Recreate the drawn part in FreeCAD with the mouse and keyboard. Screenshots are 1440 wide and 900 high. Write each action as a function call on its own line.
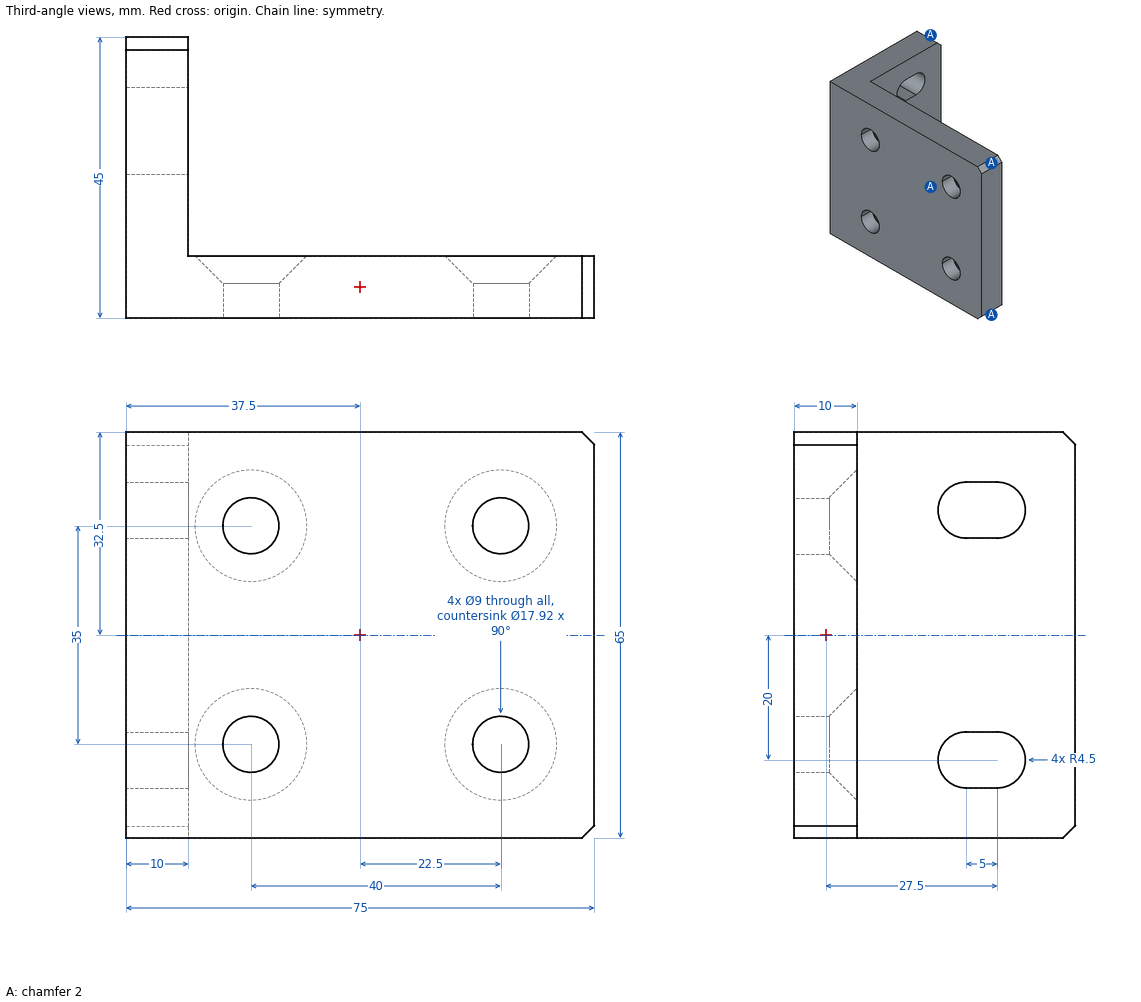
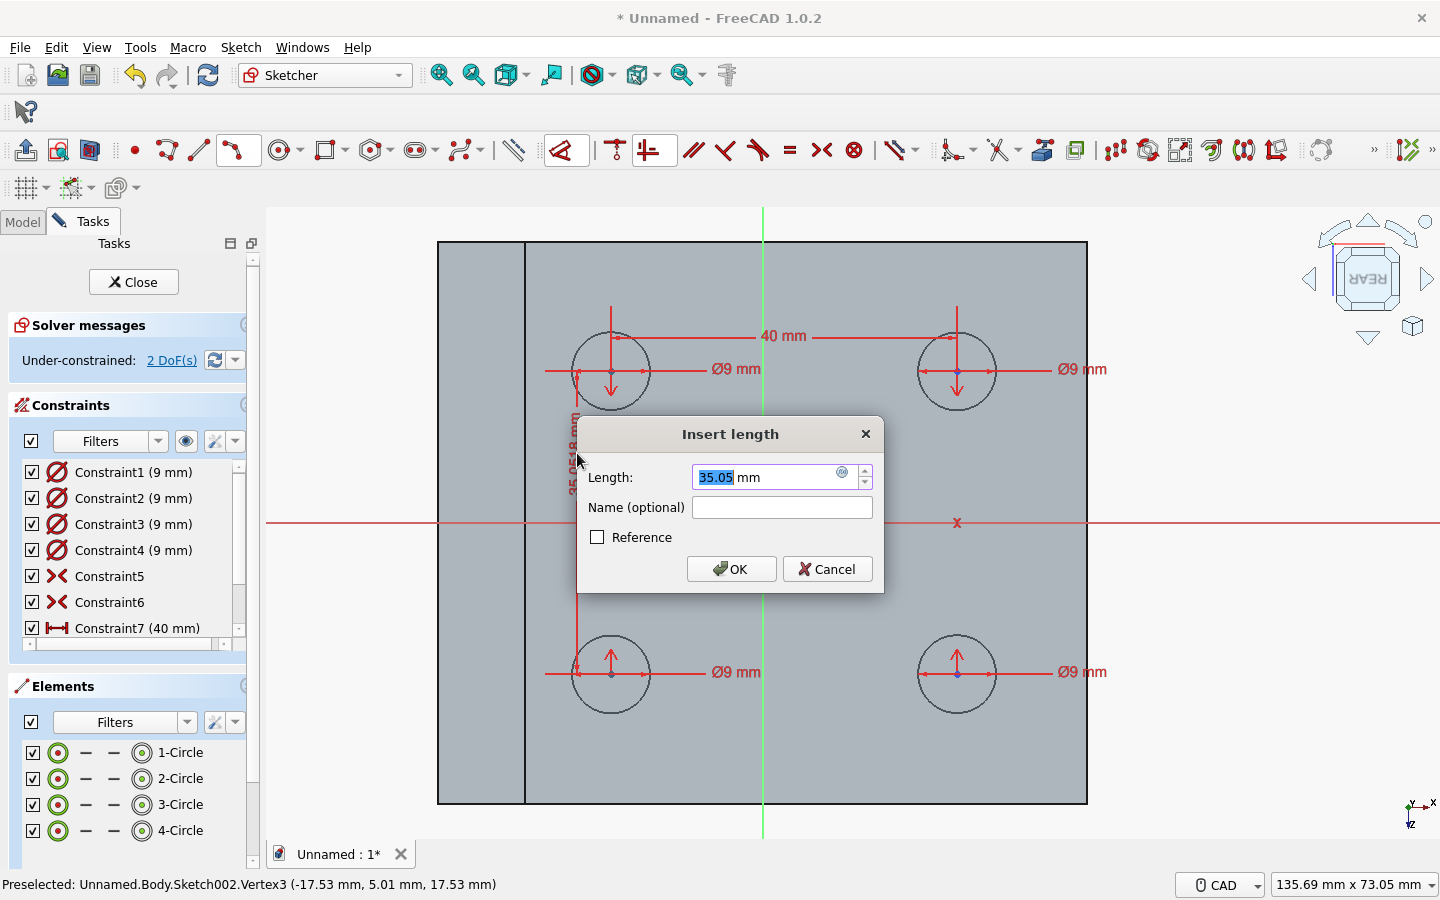
text(35)
key(Return)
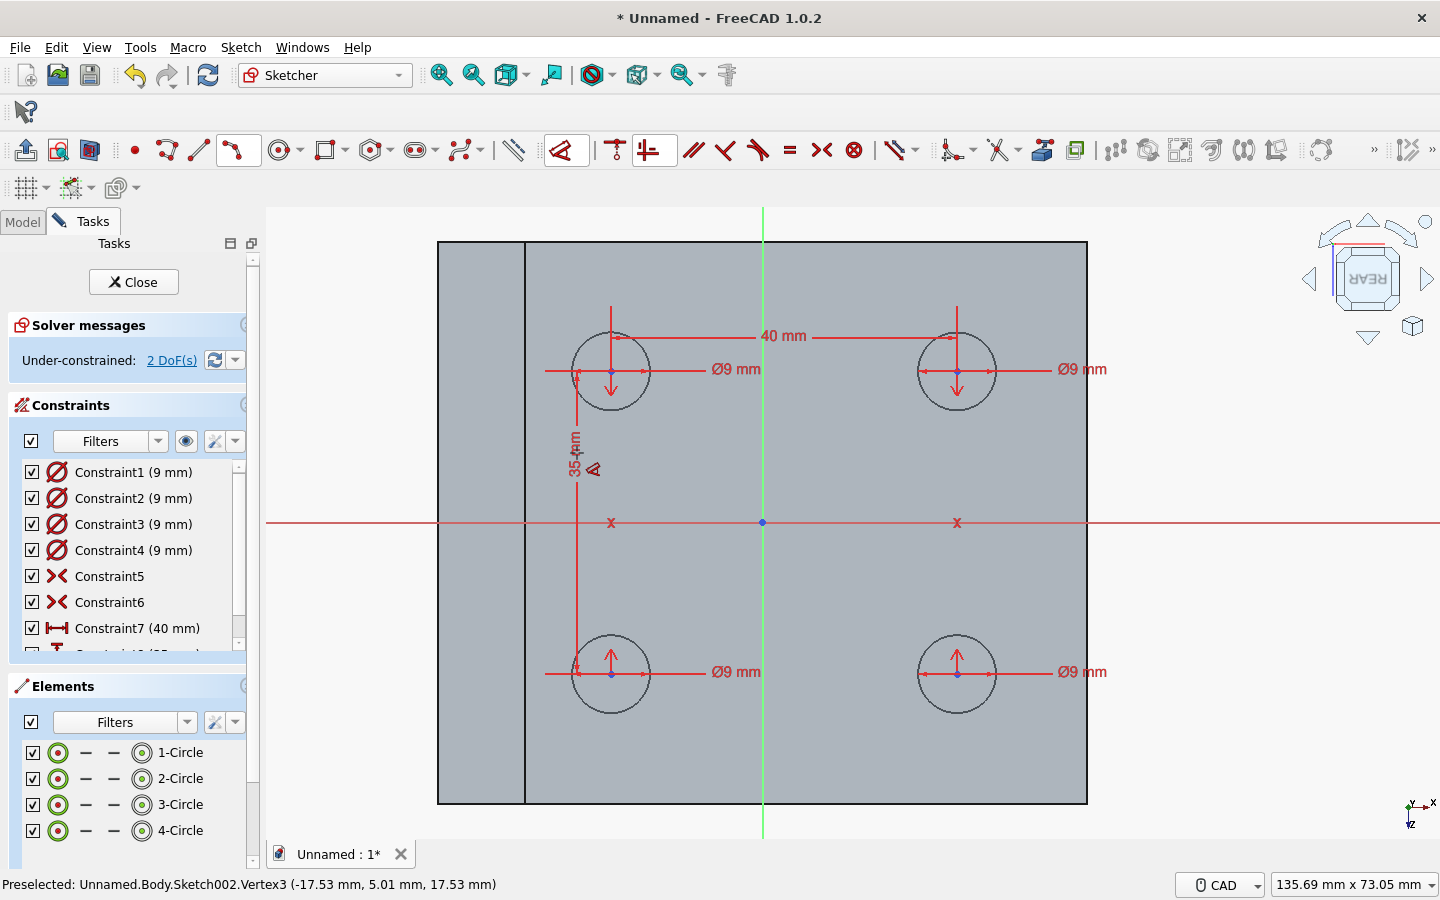
click(957, 371)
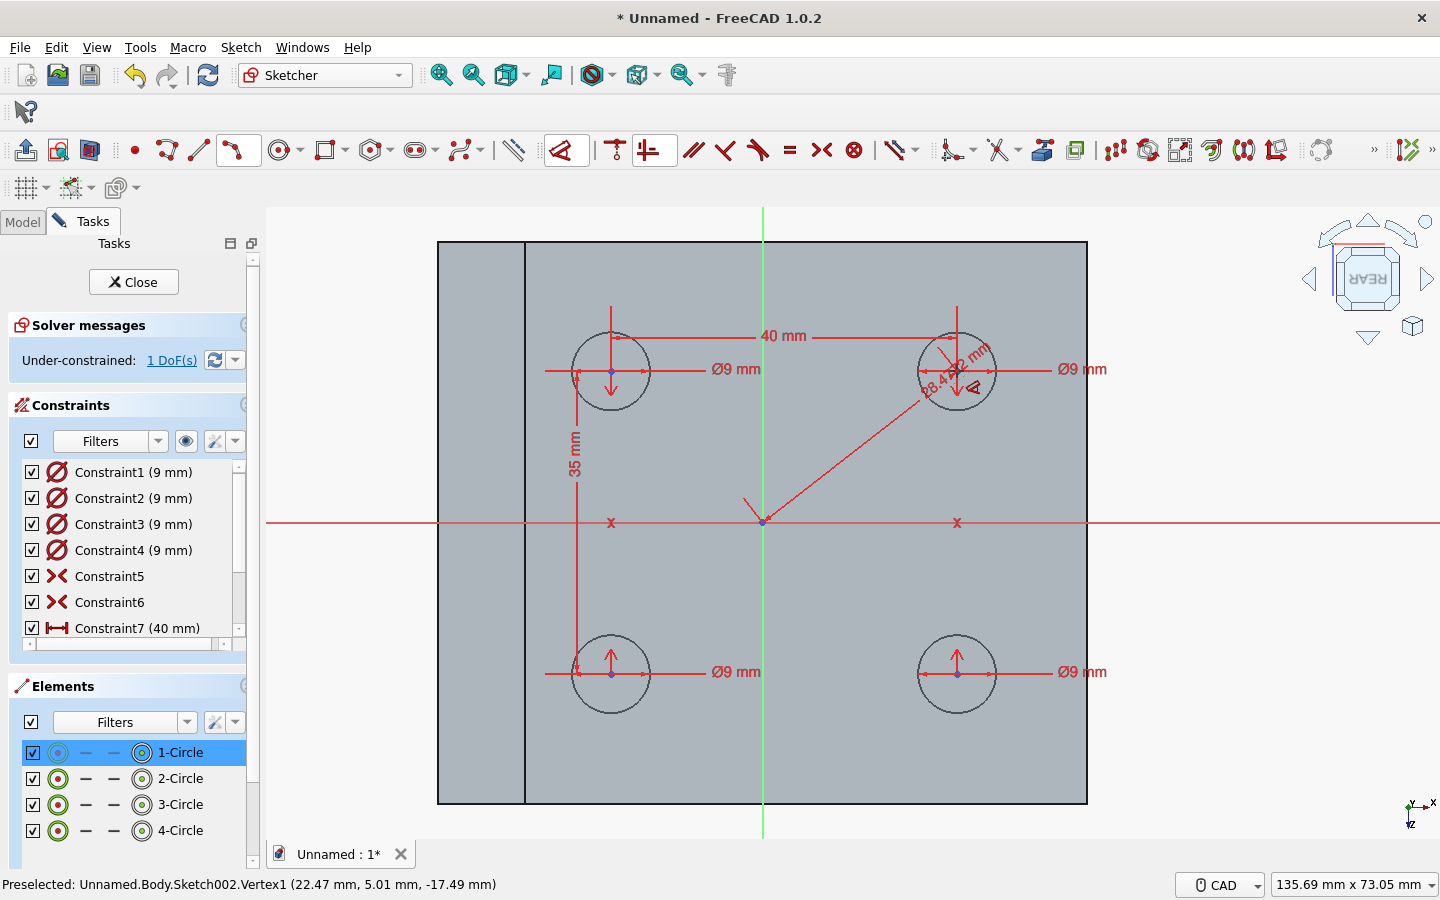
click(611, 674)
click(577, 592)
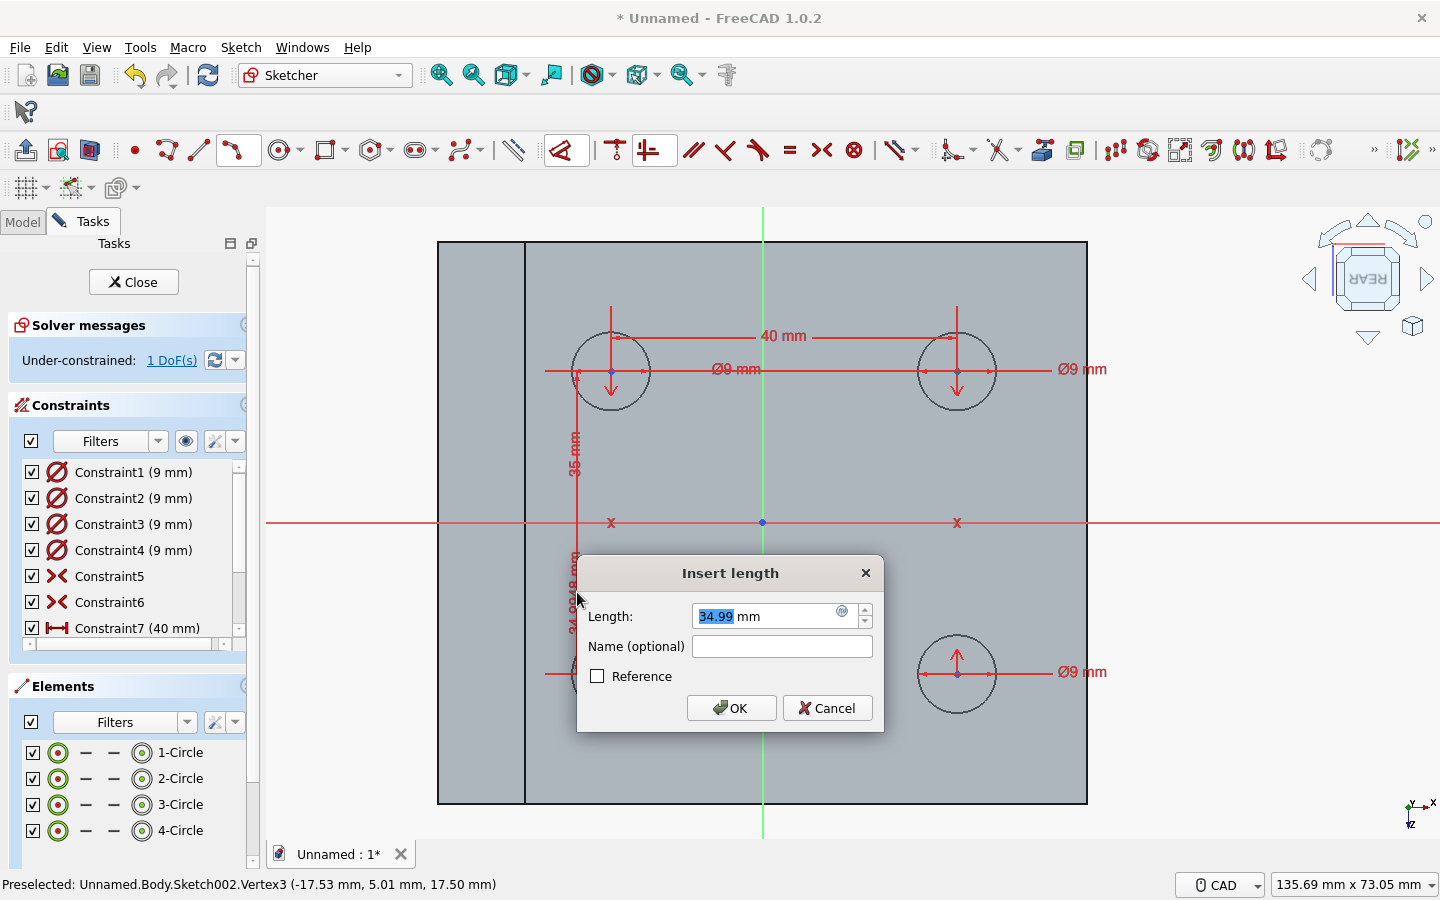
text(35)
key(Return)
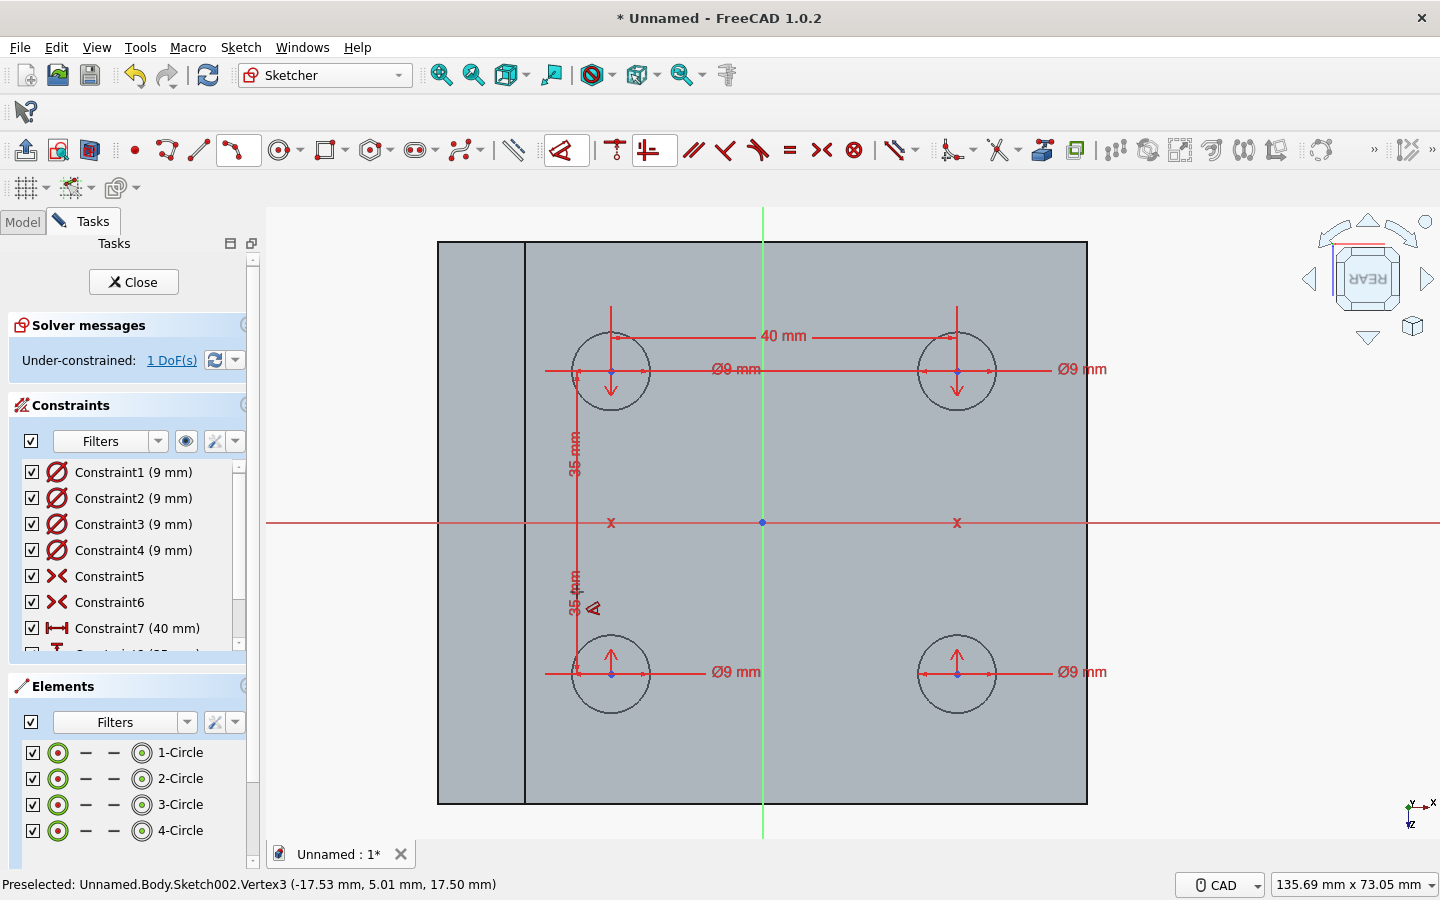
click(957, 371)
click(860, 337)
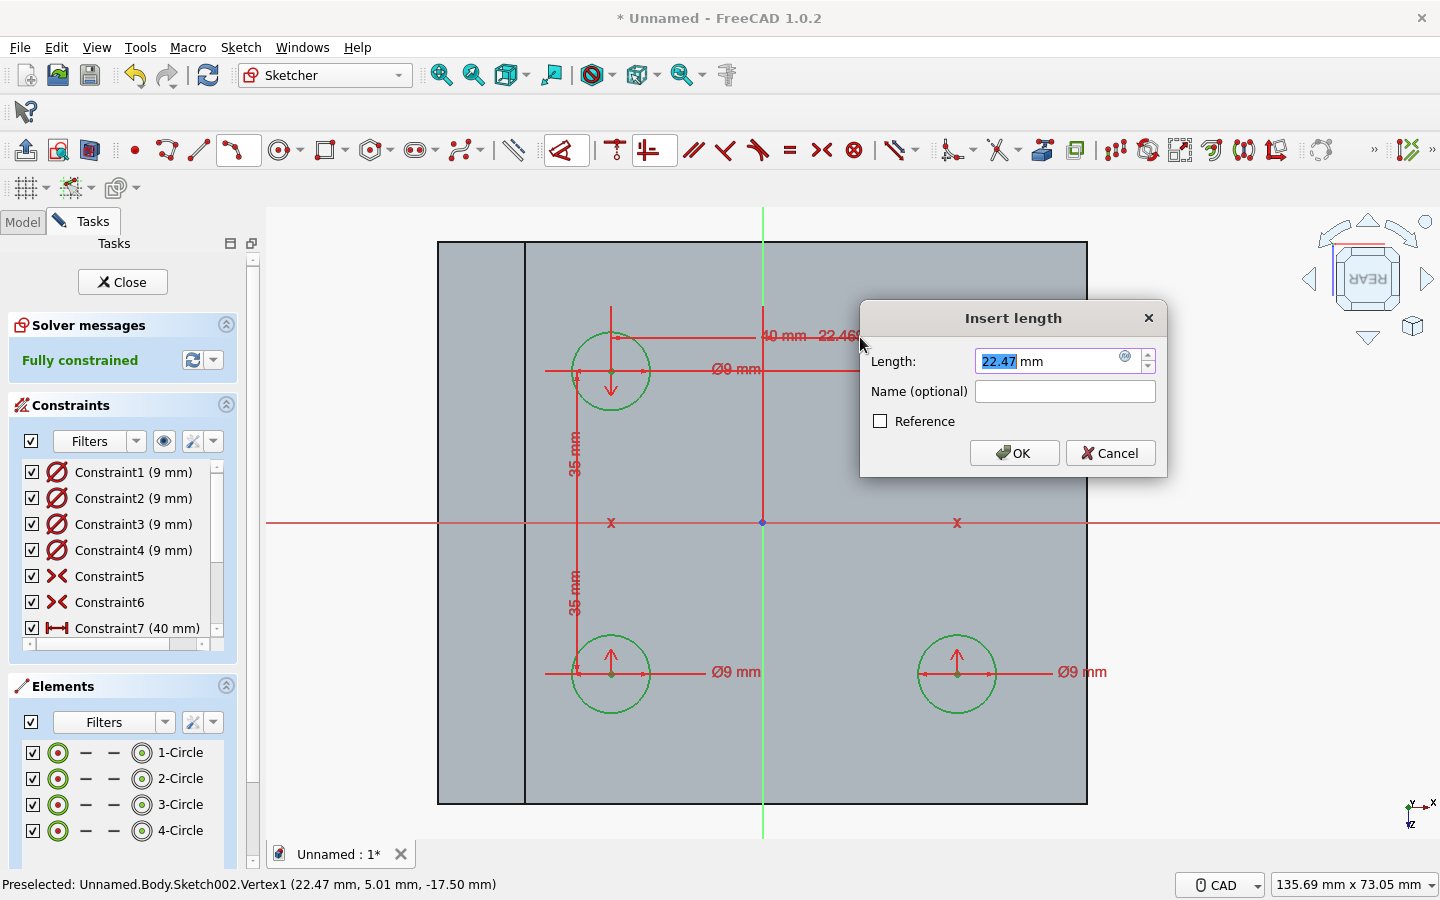
text(22.5)
key(Return)
key(Escape)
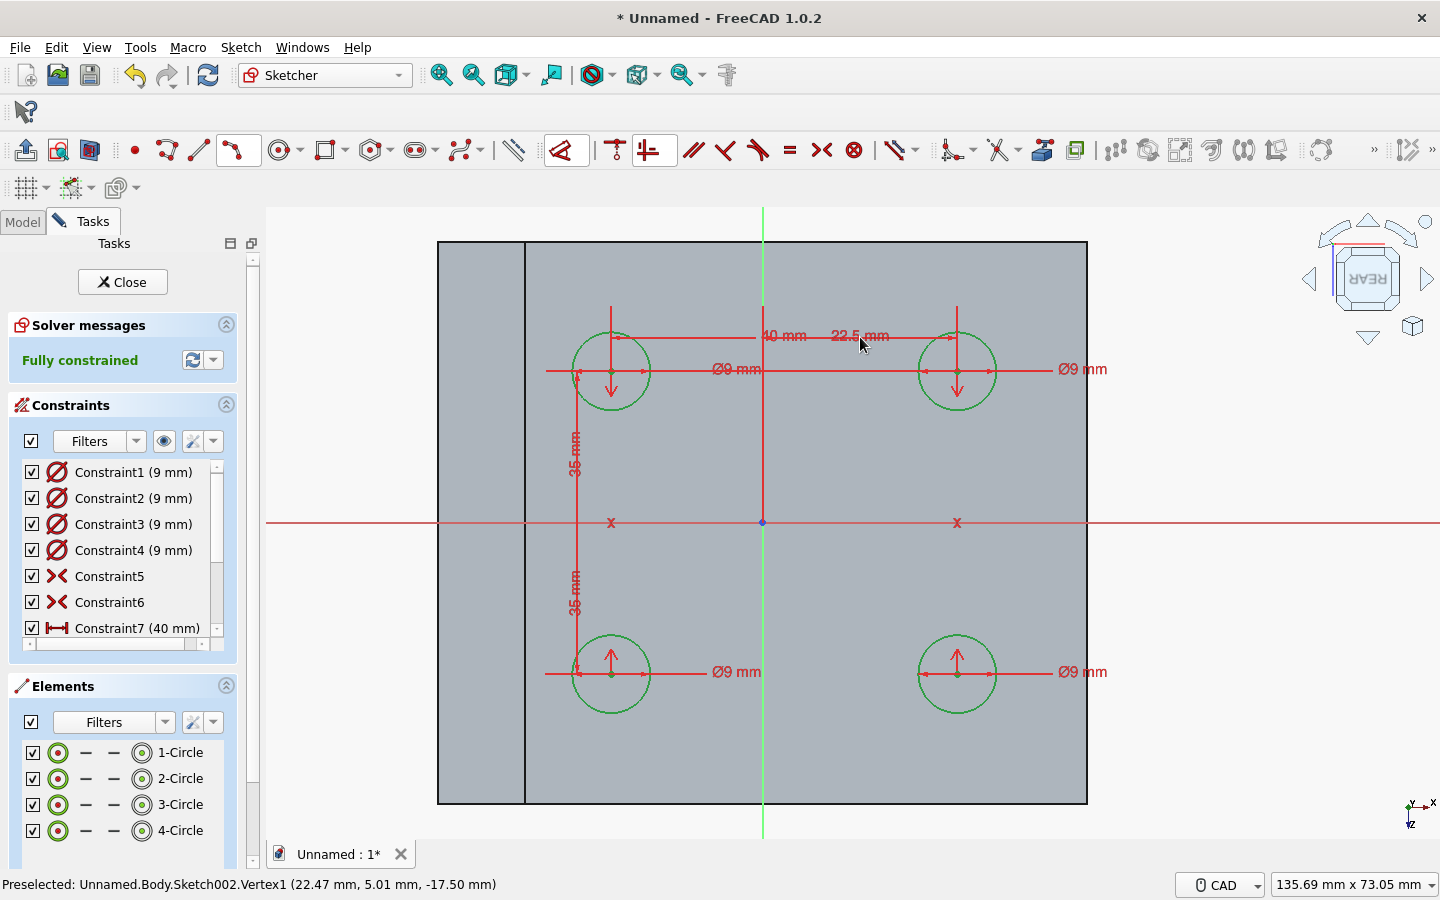
click(123, 282)